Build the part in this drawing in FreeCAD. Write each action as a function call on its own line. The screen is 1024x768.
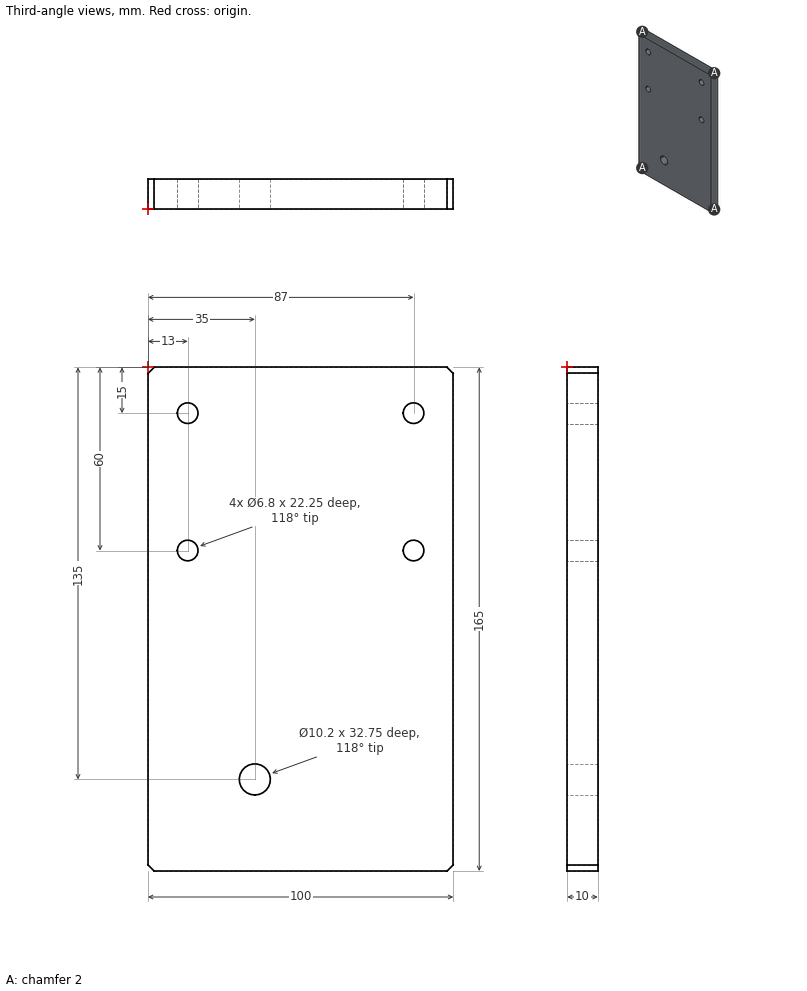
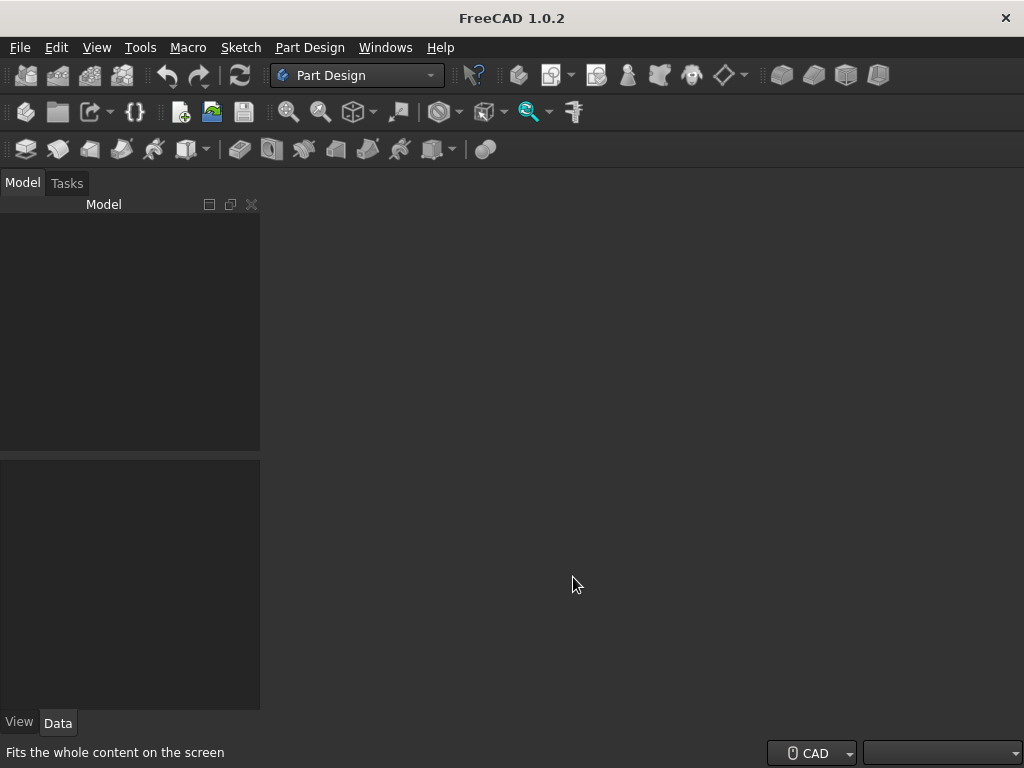
click(180, 112)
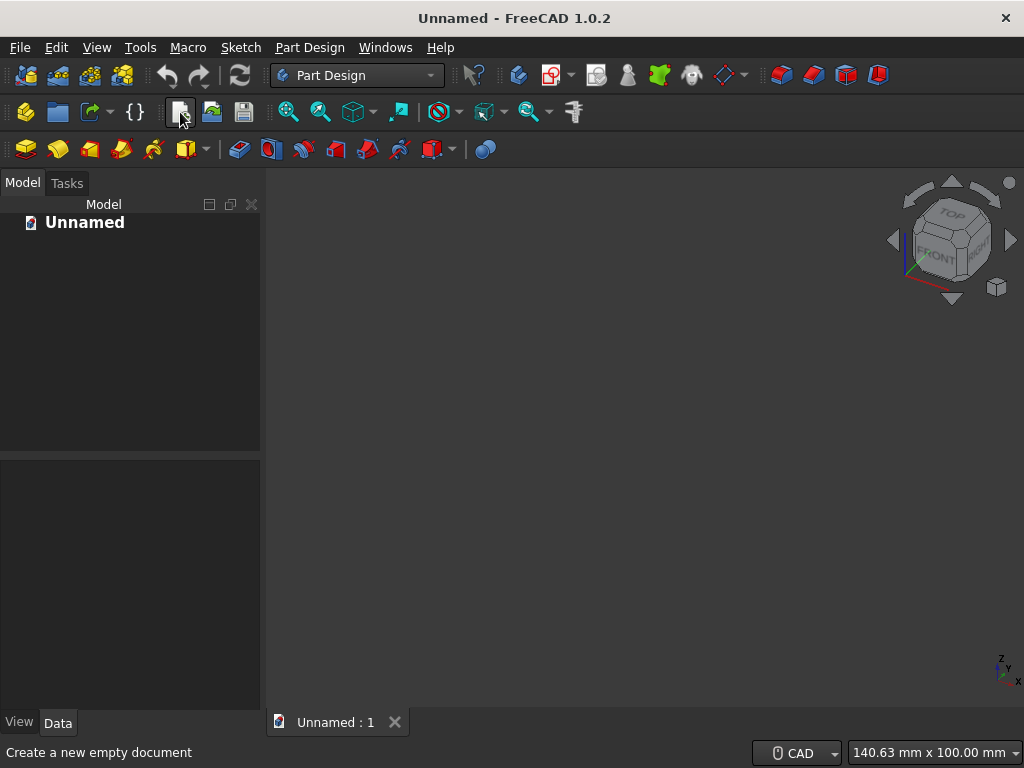
click(552, 76)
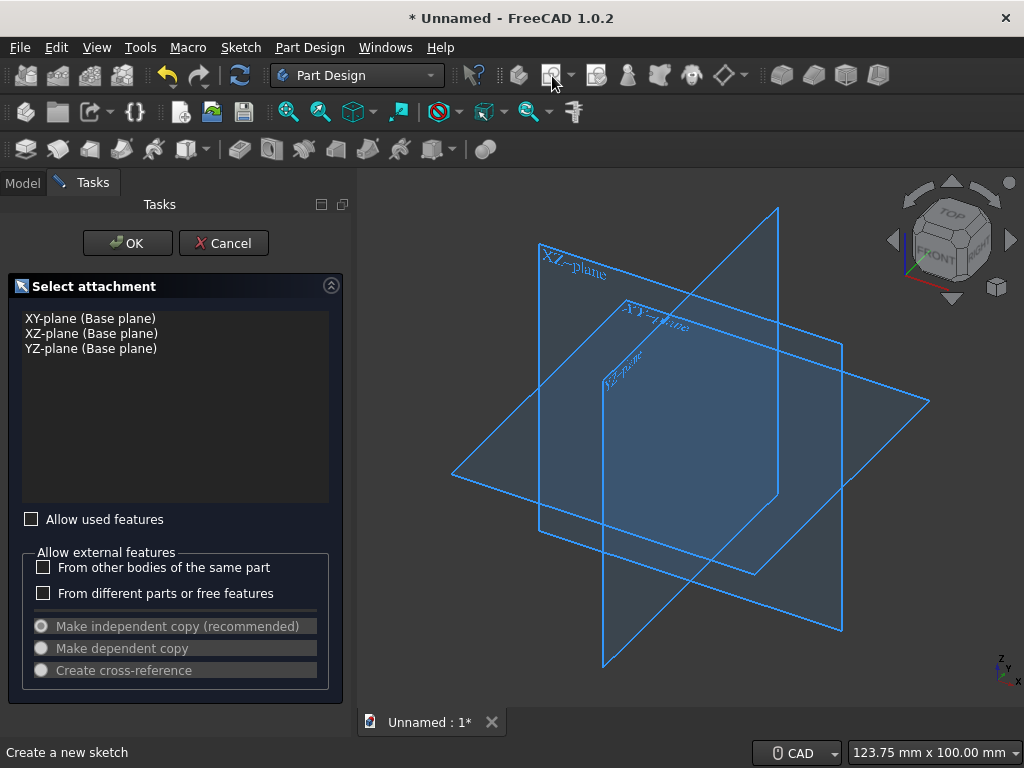
click(82, 334)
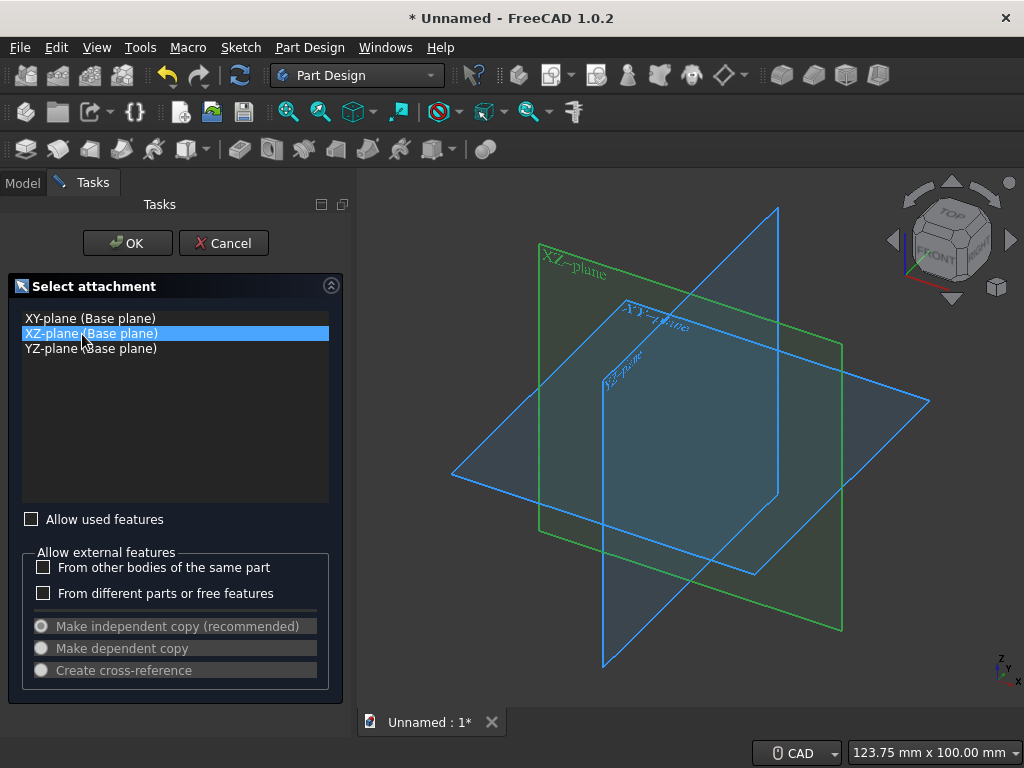
click(128, 243)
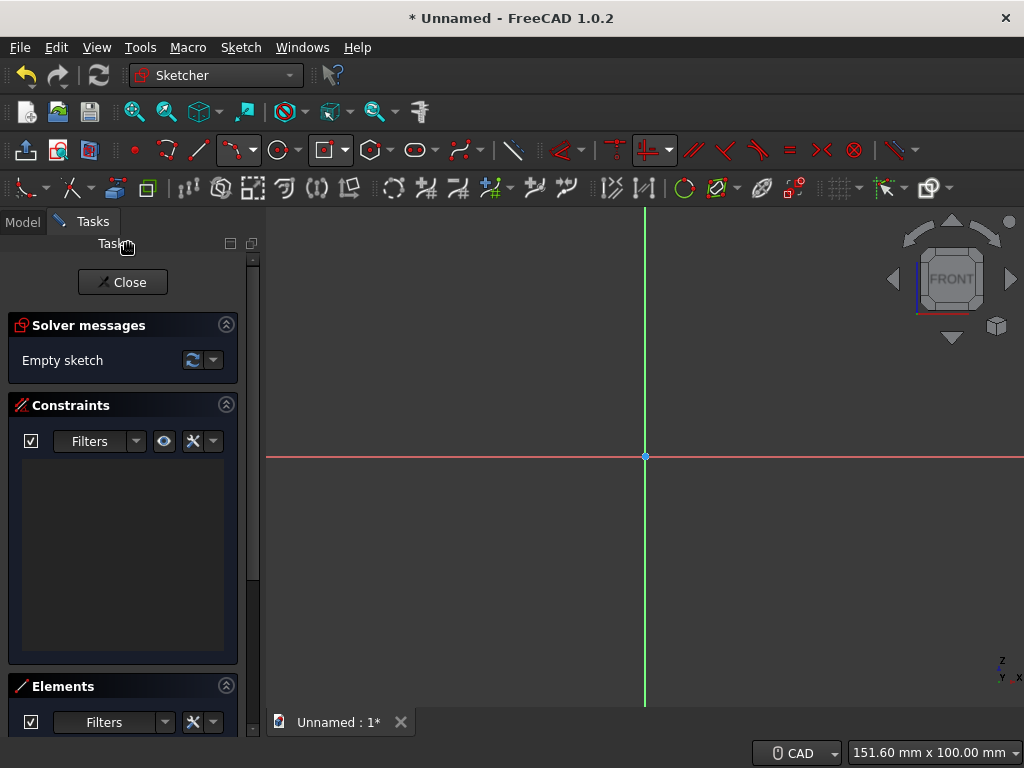
scroll(391, 235, down, 5)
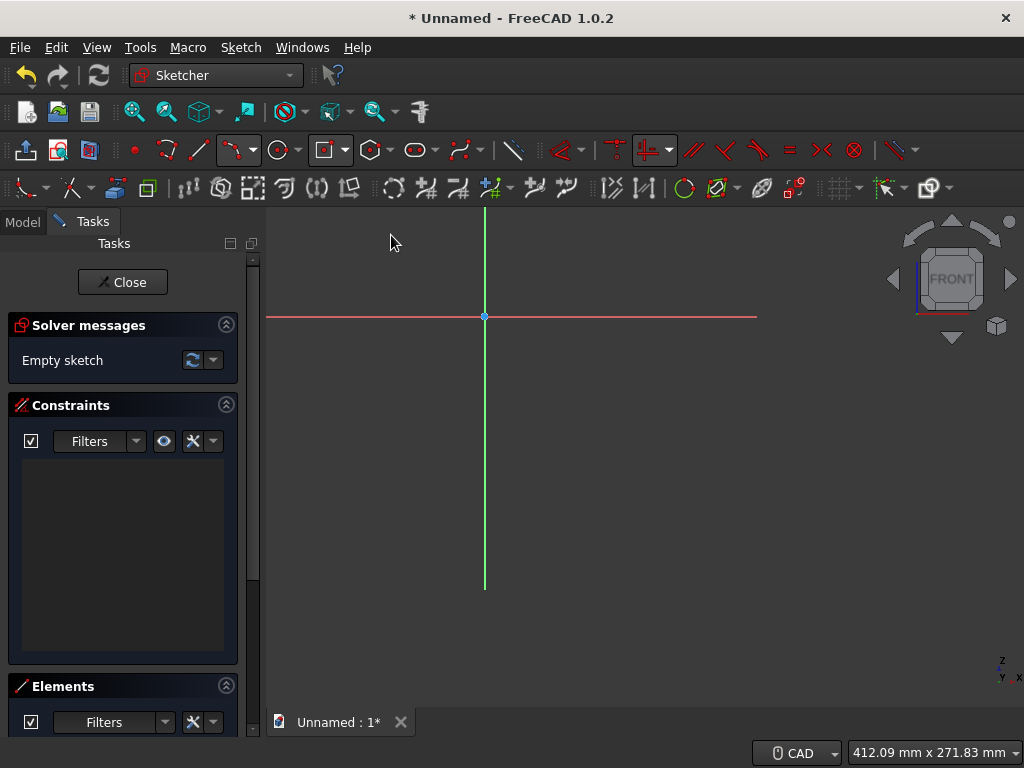
key(g)
key(r)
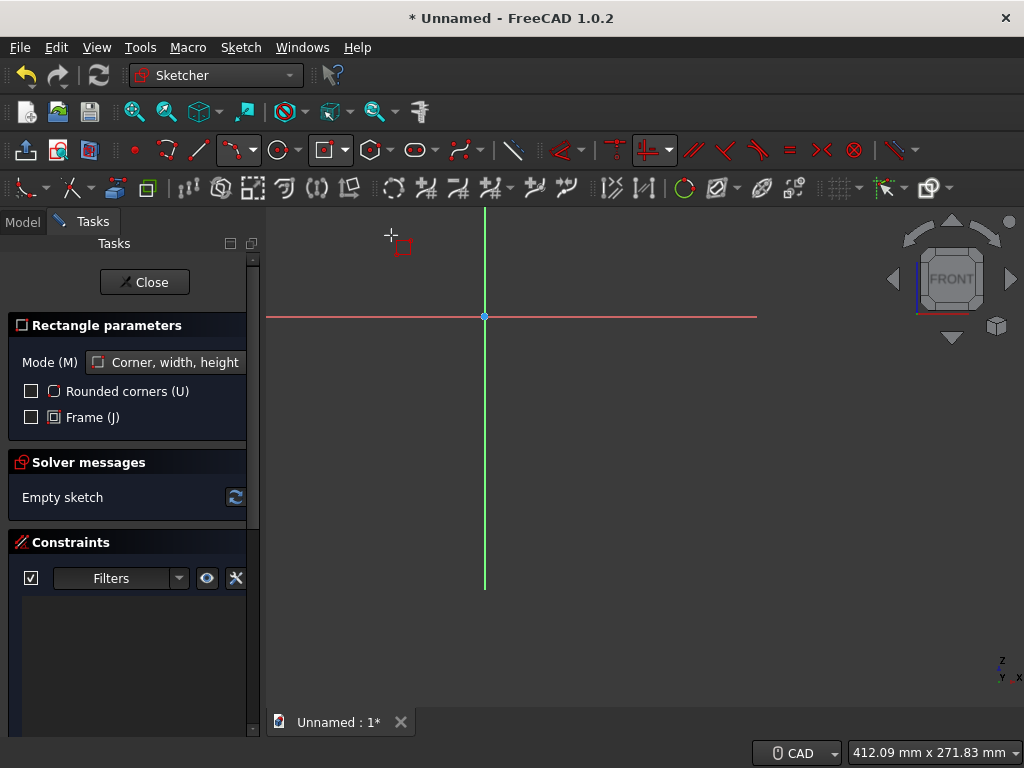
click(485, 317)
move(668, 620)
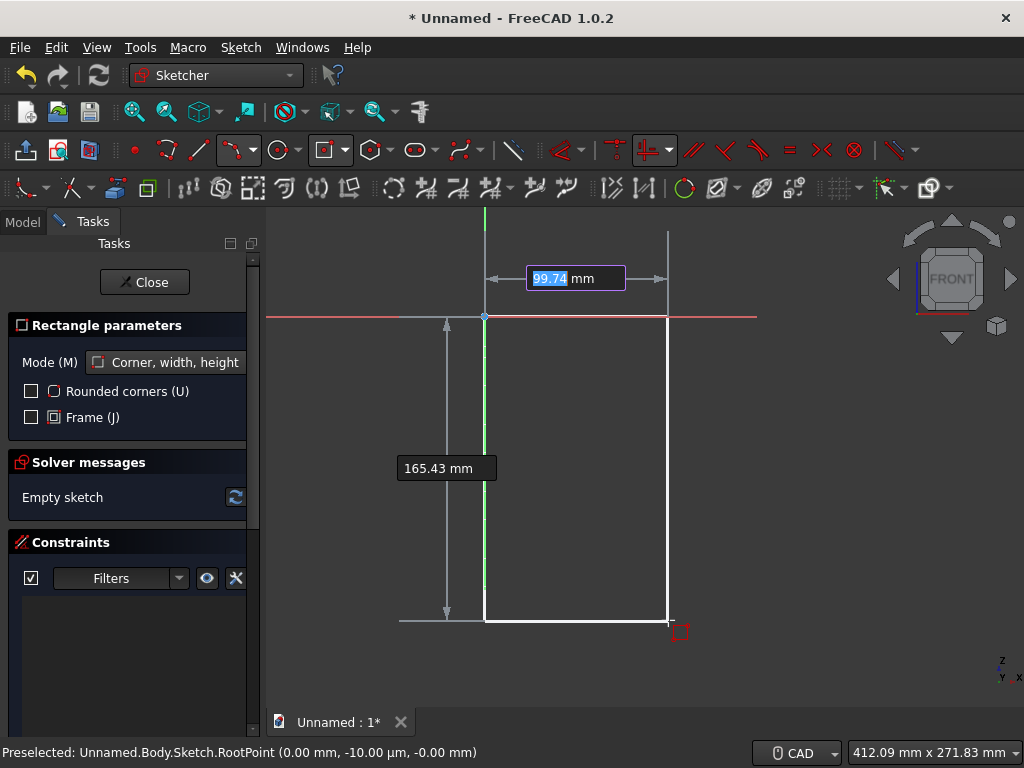
text(100)
key(Tab)
text(165)
key(Return)
key(Escape)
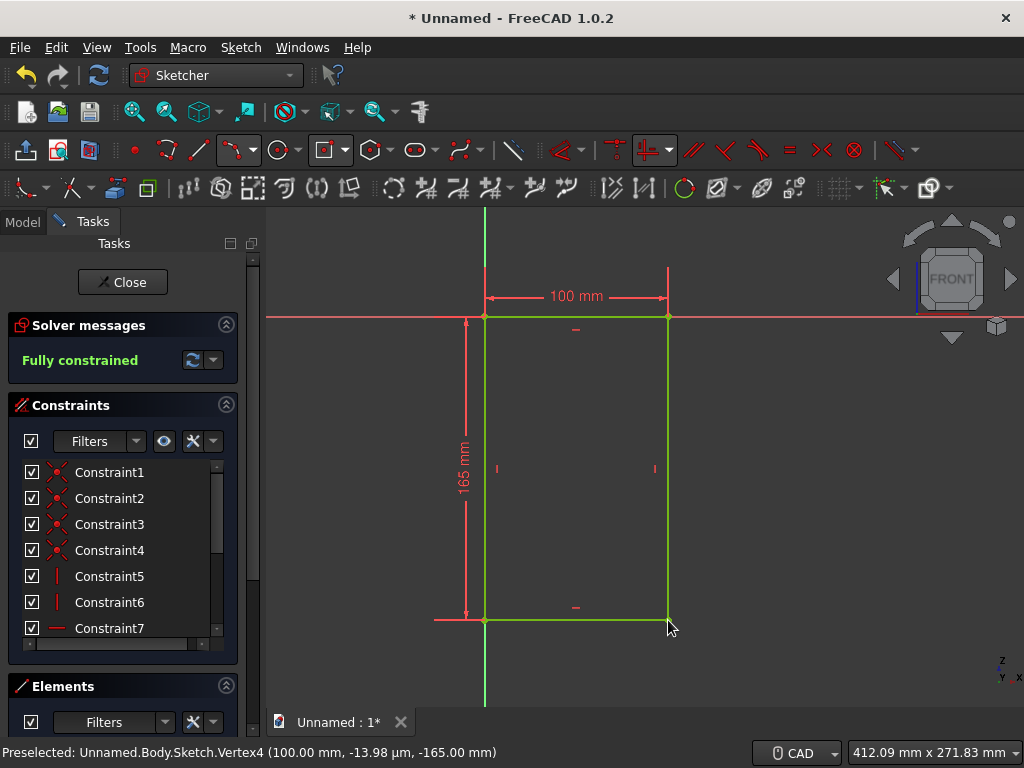
click(123, 282)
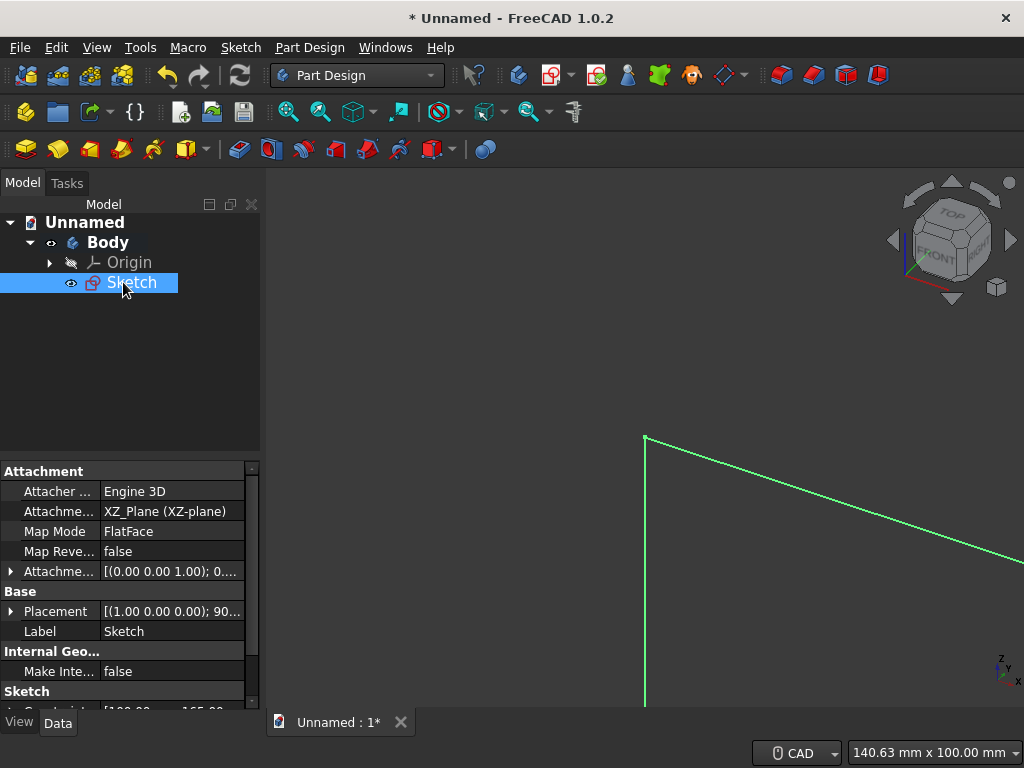
click(26, 150)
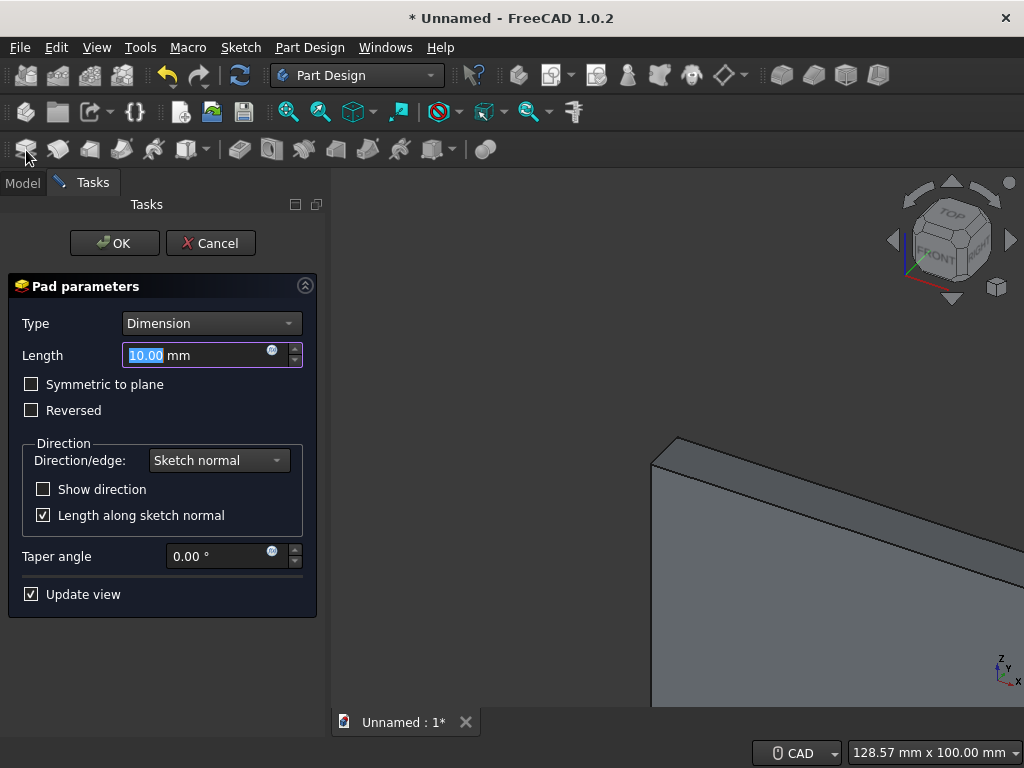
text(10)
key(Tab)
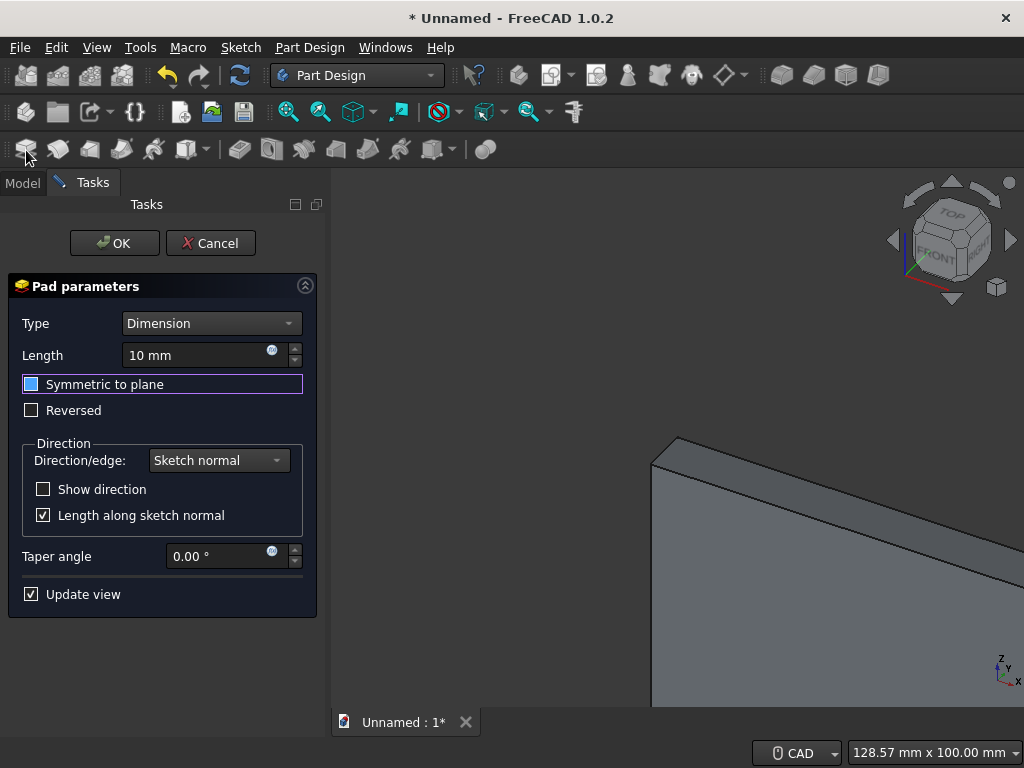
click(30, 410)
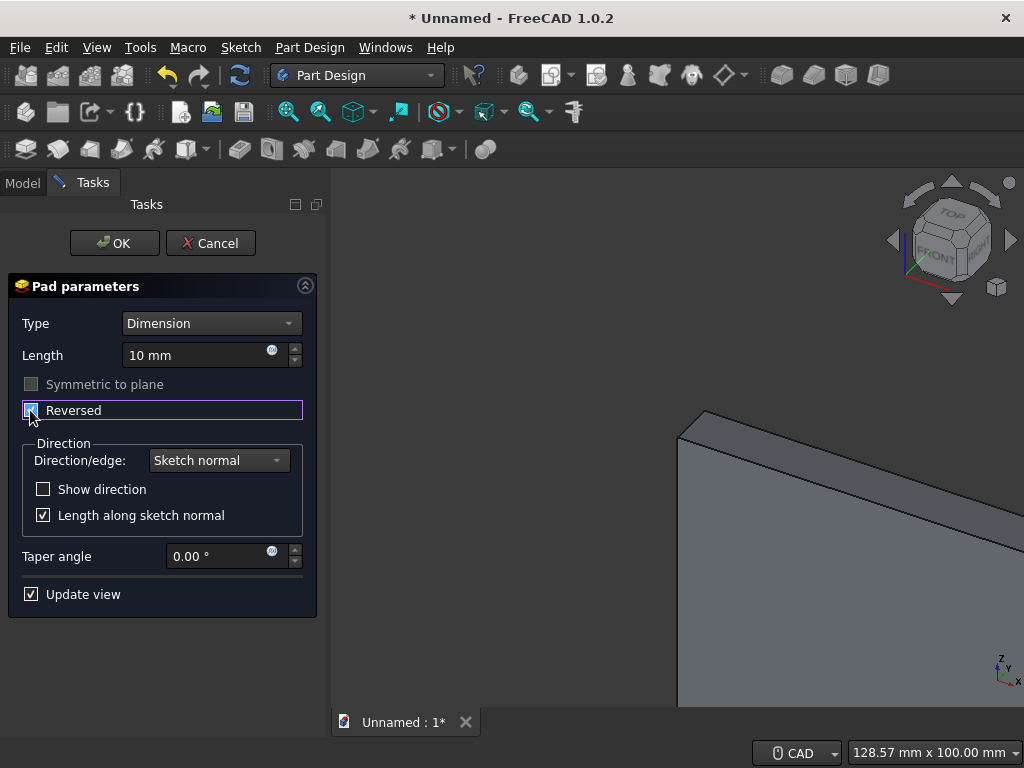
click(115, 243)